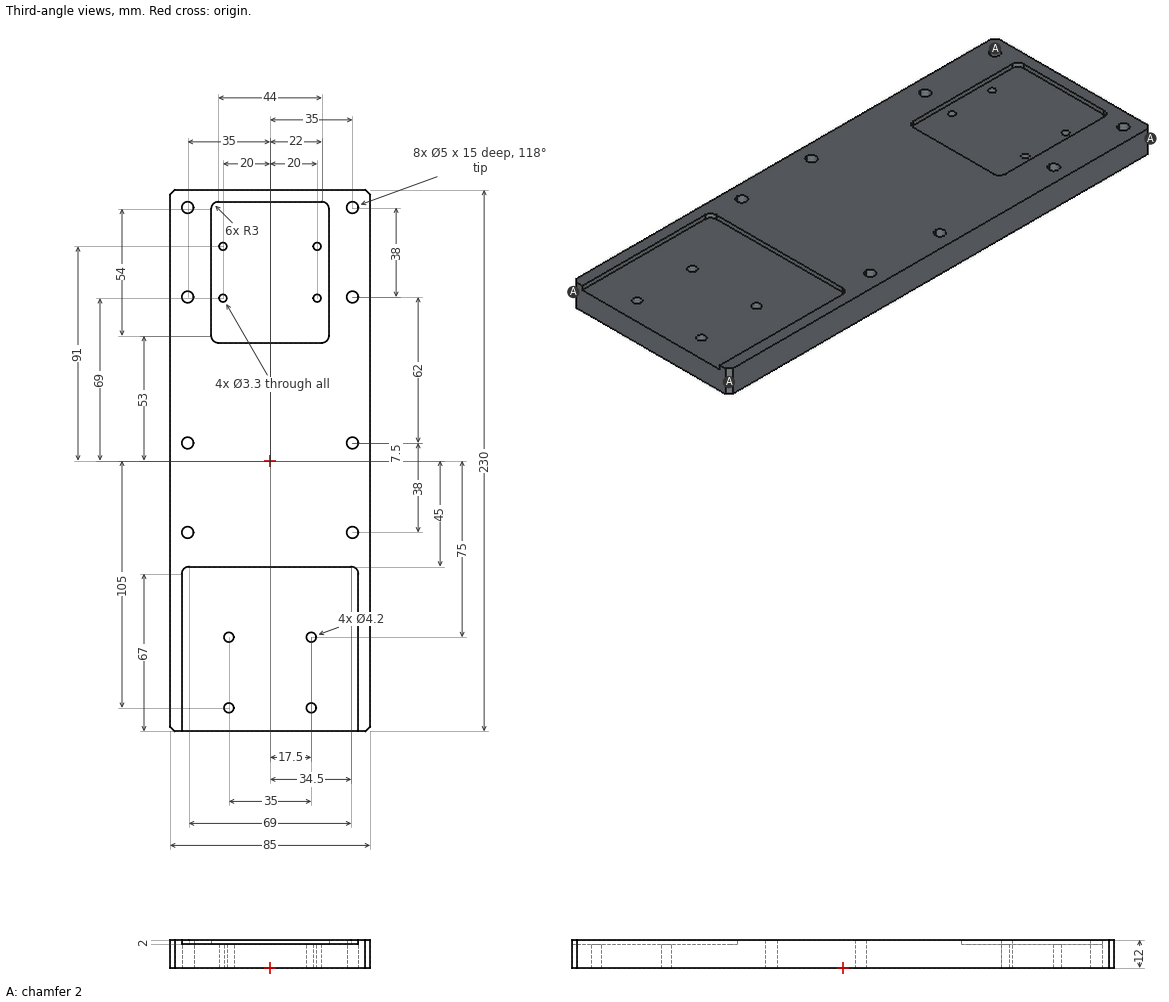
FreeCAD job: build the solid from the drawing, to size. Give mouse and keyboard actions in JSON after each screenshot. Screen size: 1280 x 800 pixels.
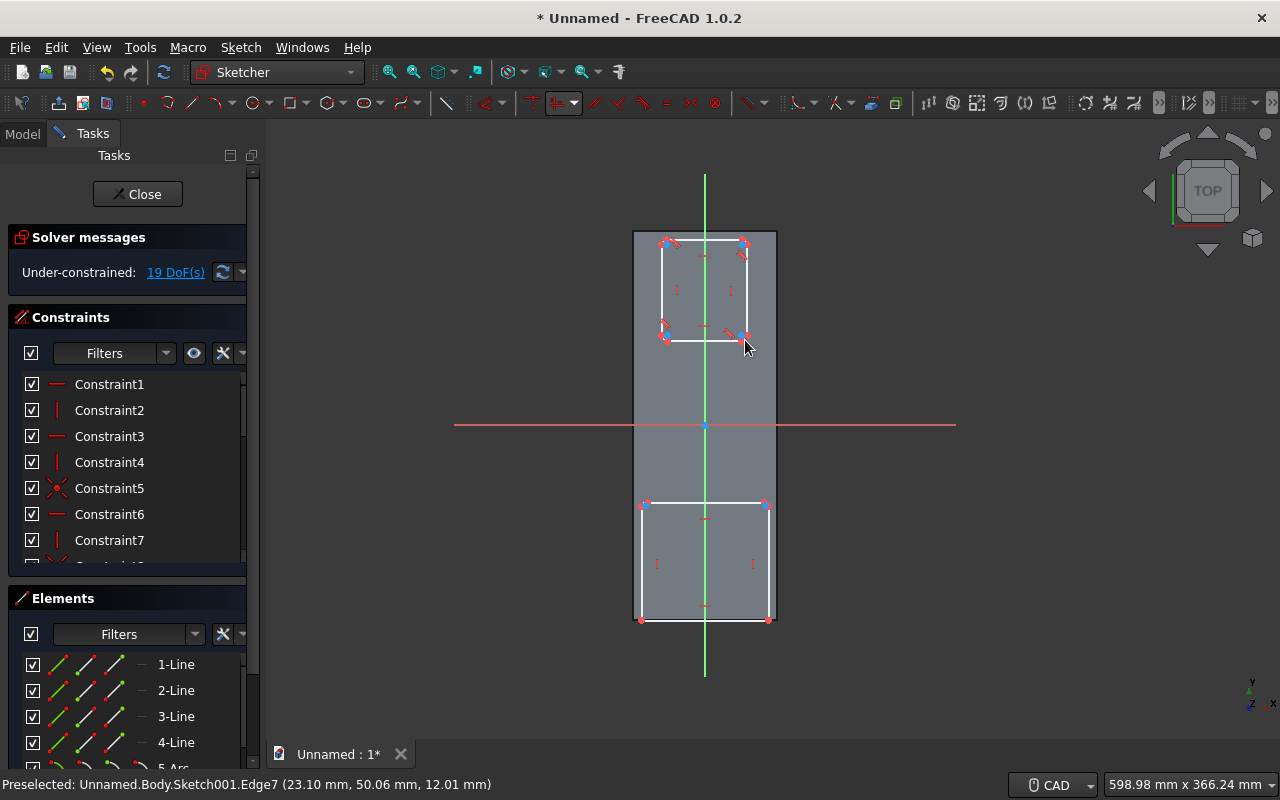
{"action": "left_click", "coordinate": [747, 308]}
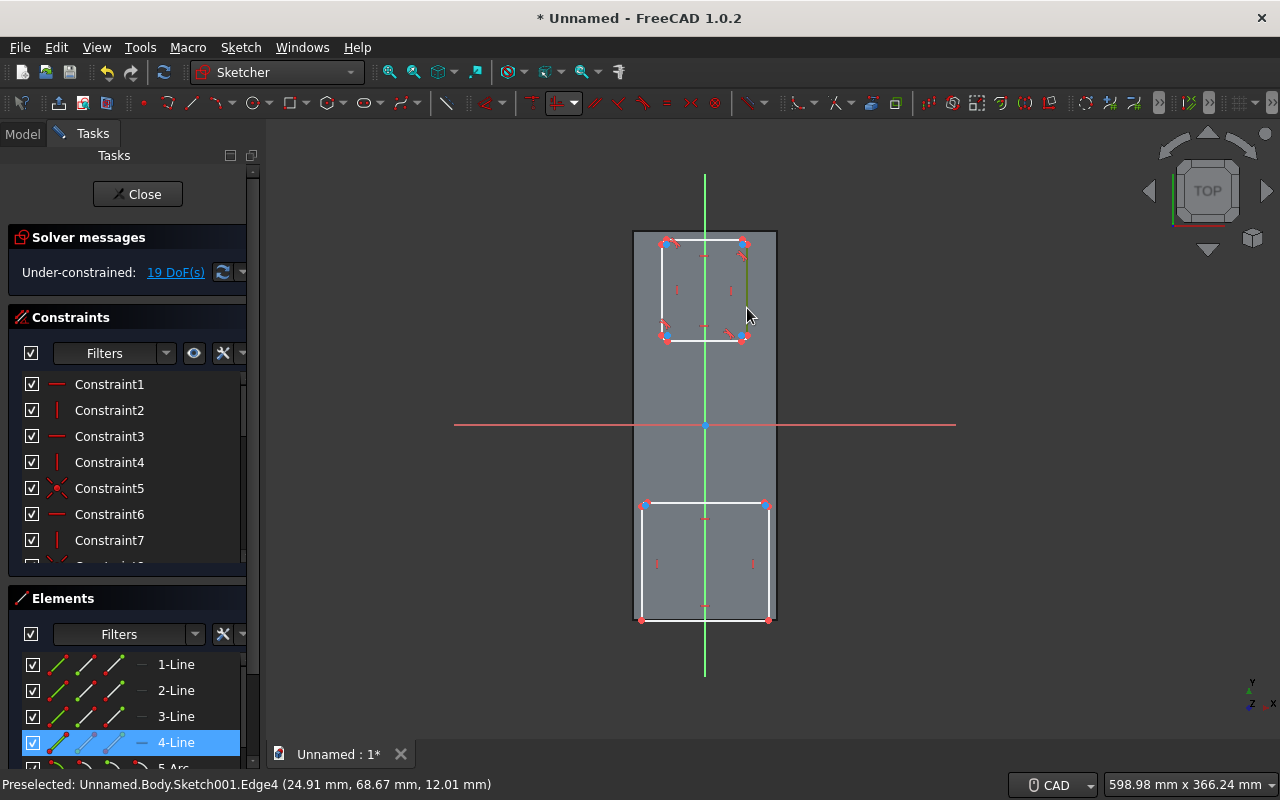
{"action": "scroll", "coordinate": [746, 241], "scroll_direction": "up", "scroll_amount": 7}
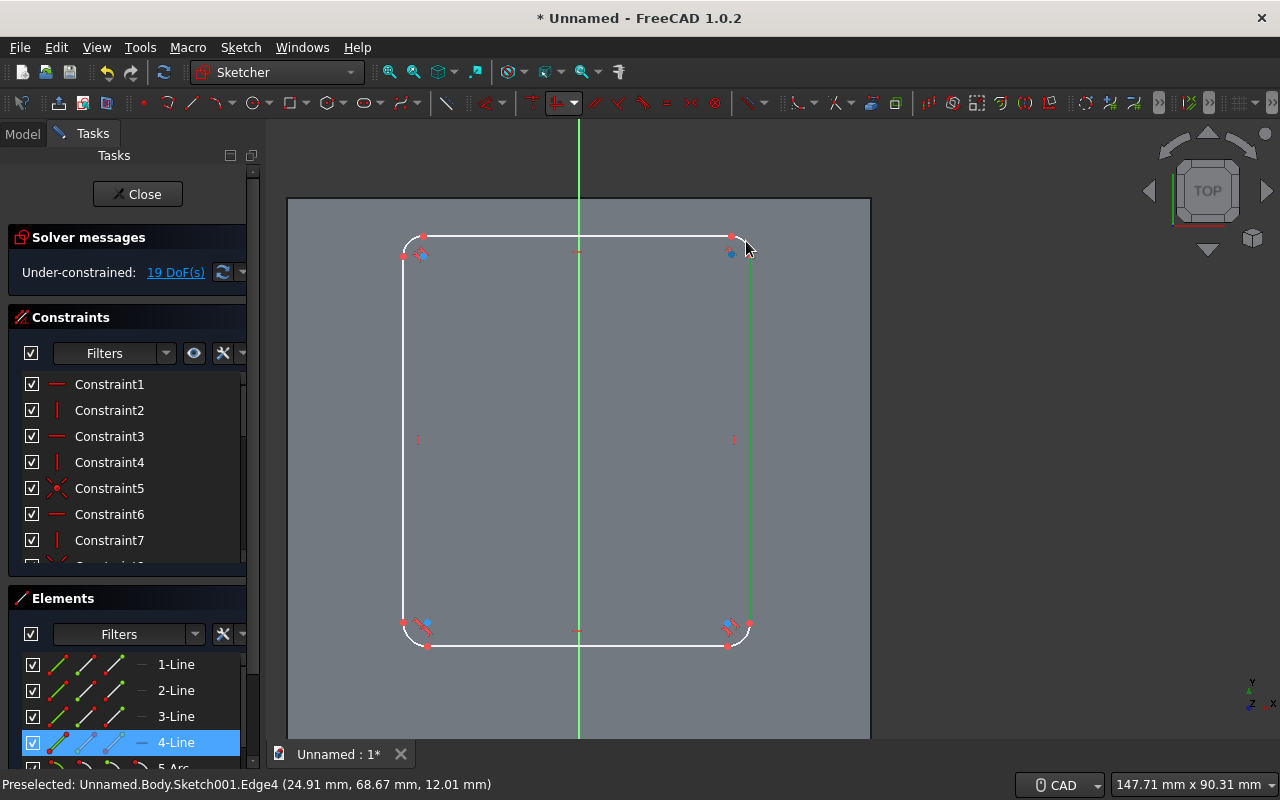
{"action": "left_click", "coordinate": [744, 242]}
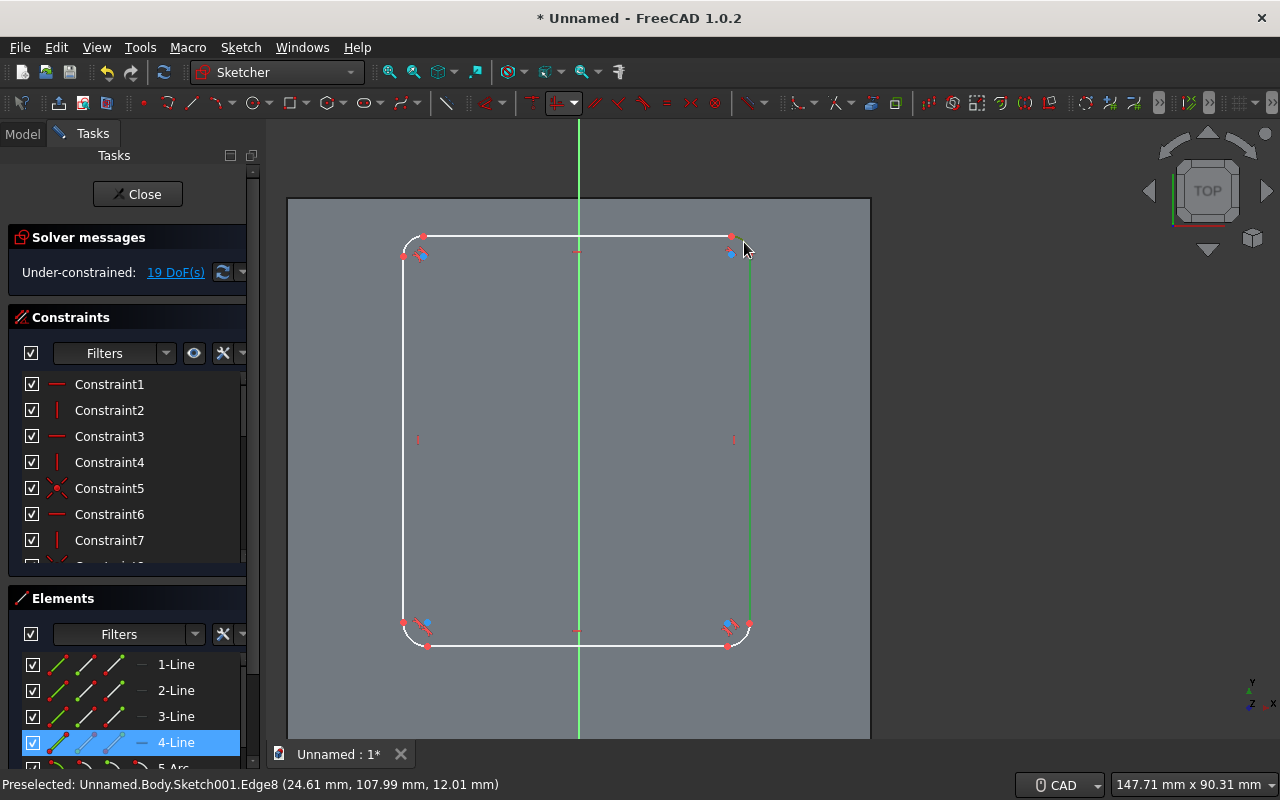
{"action": "left_click", "coordinate": [644, 104]}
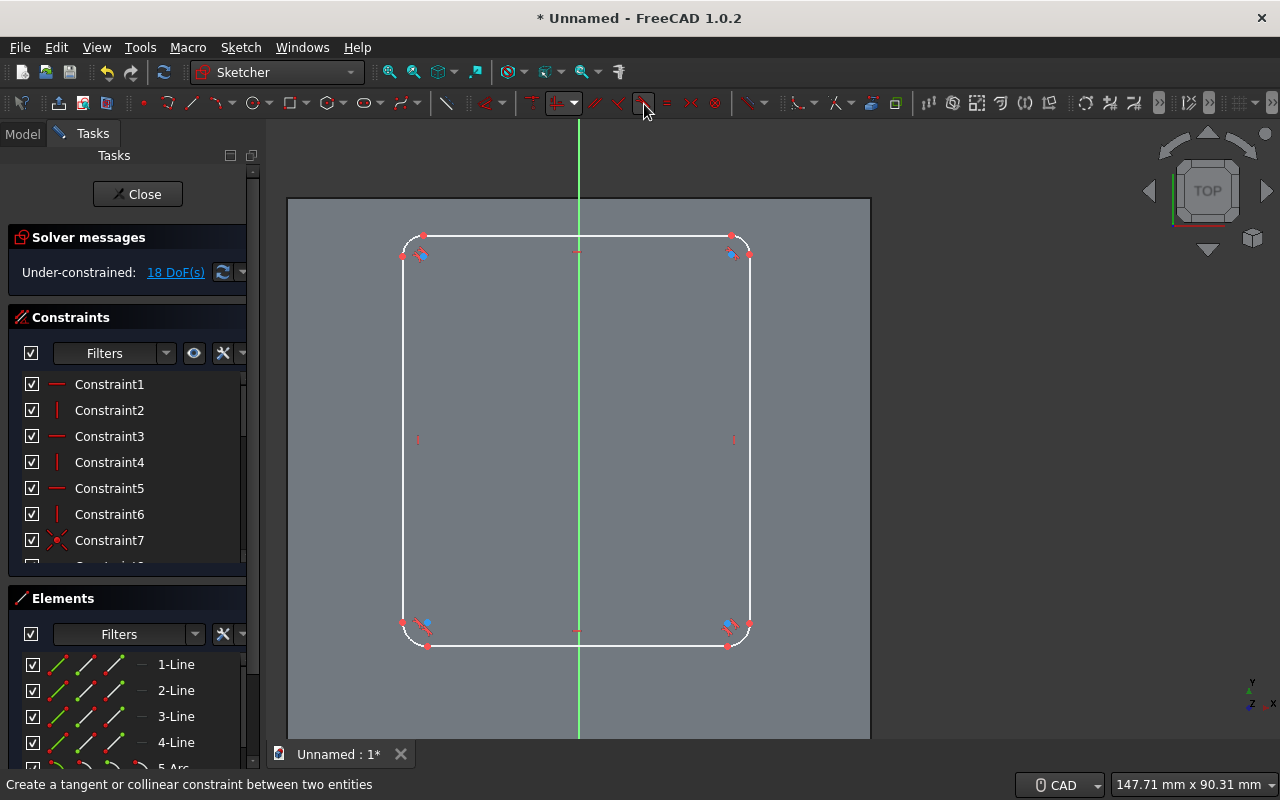
{"action": "scroll", "coordinate": [746, 241], "scroll_direction": "down", "scroll_amount": 7}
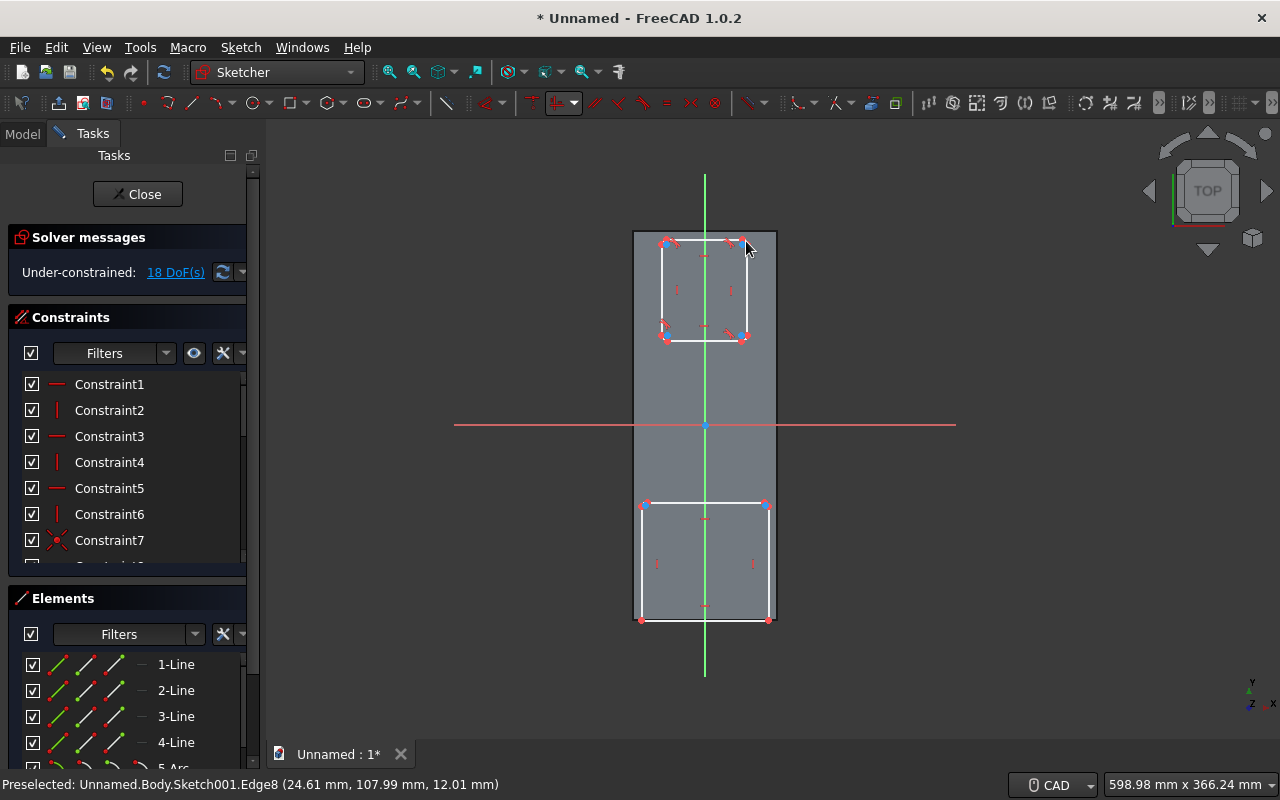
{"action": "left_click", "coordinate": [729, 503]}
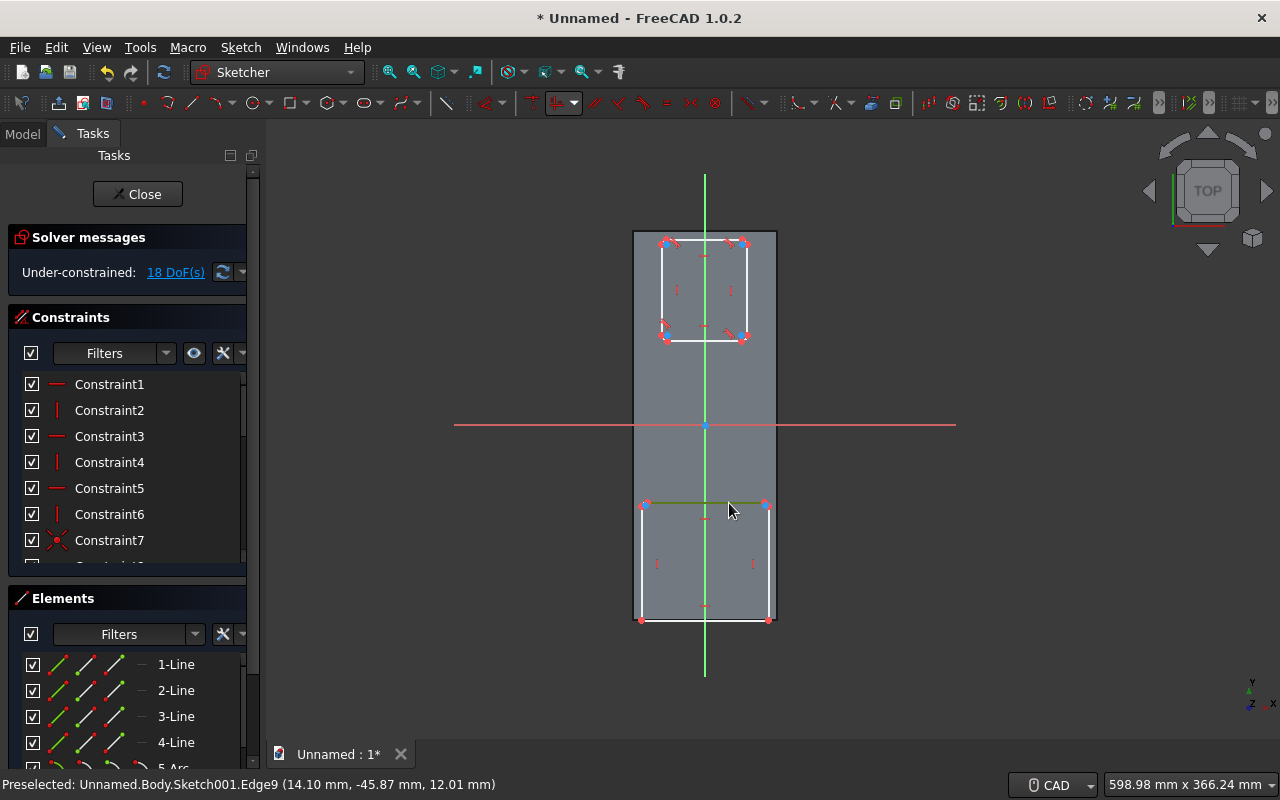
{"action": "scroll", "coordinate": [643, 503], "scroll_direction": "up", "scroll_amount": 7}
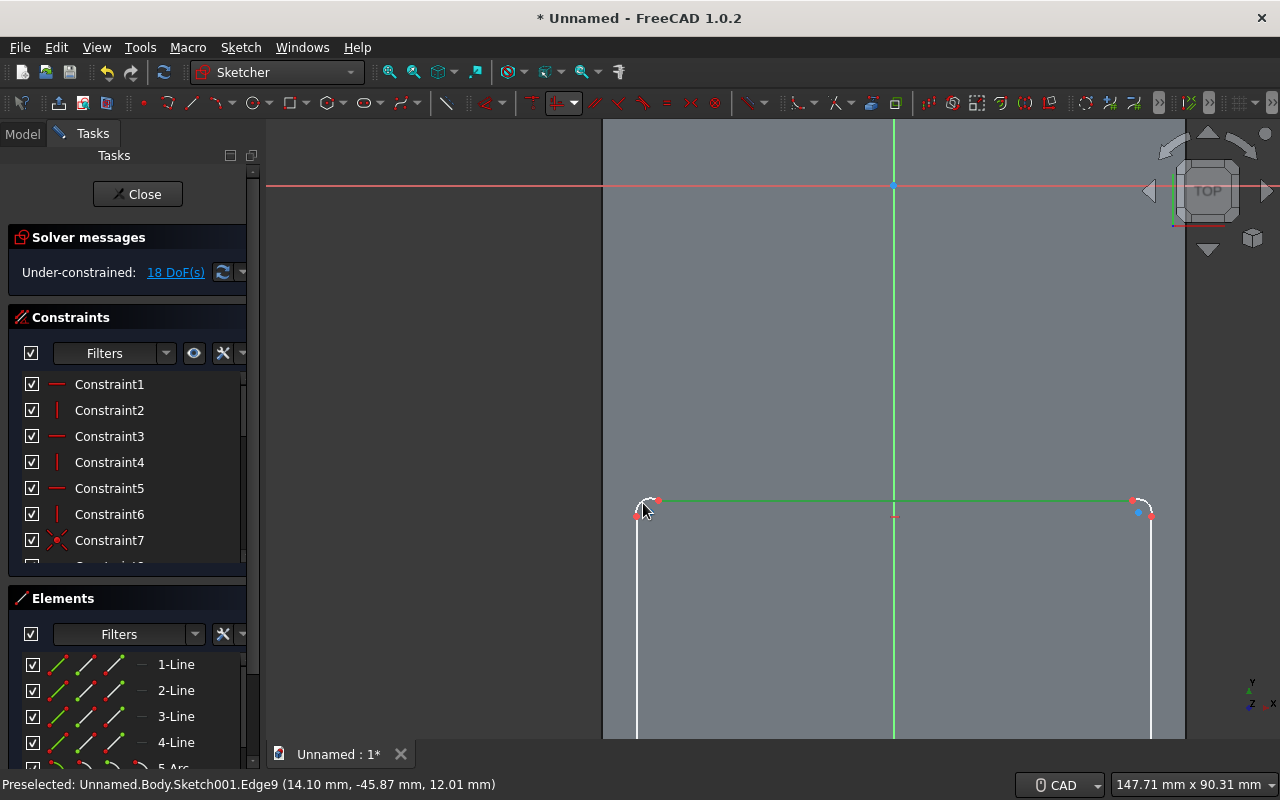
{"action": "left_click", "coordinate": [642, 501]}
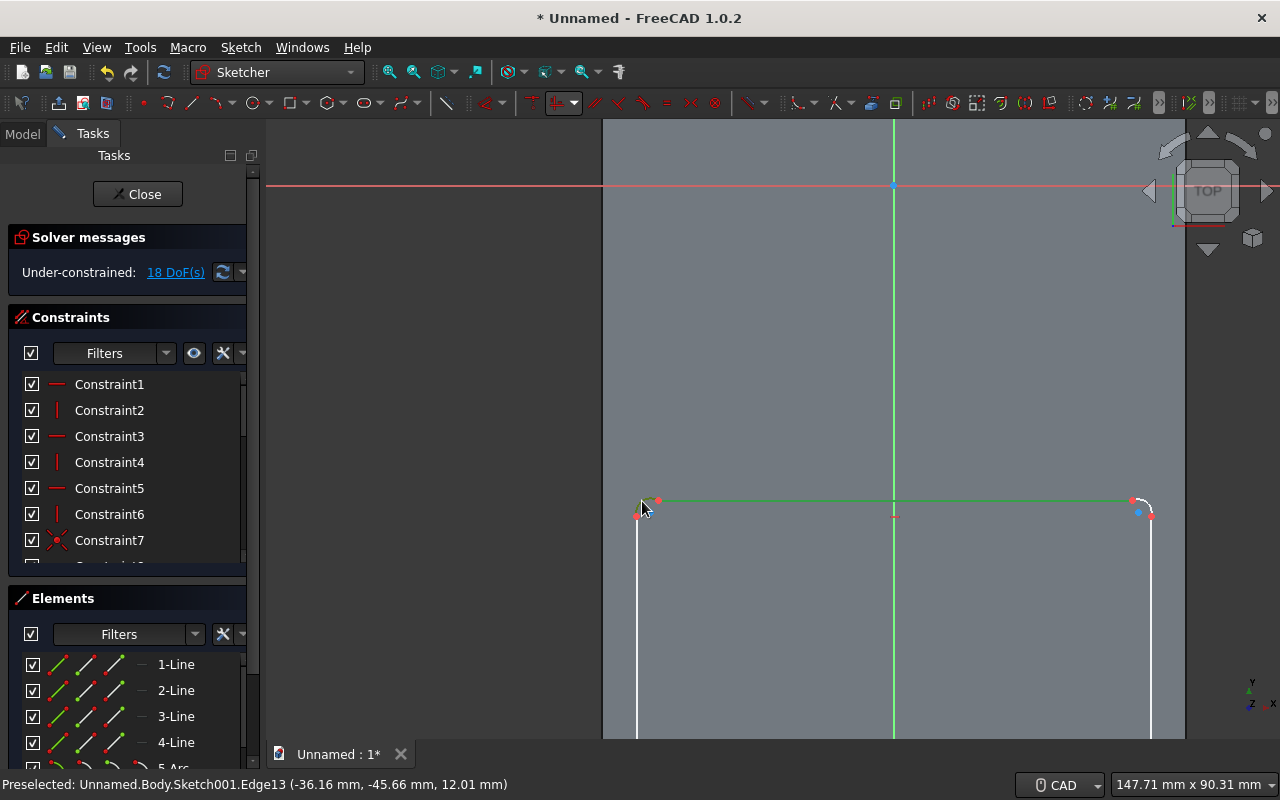
{"action": "key", "text": "t"}